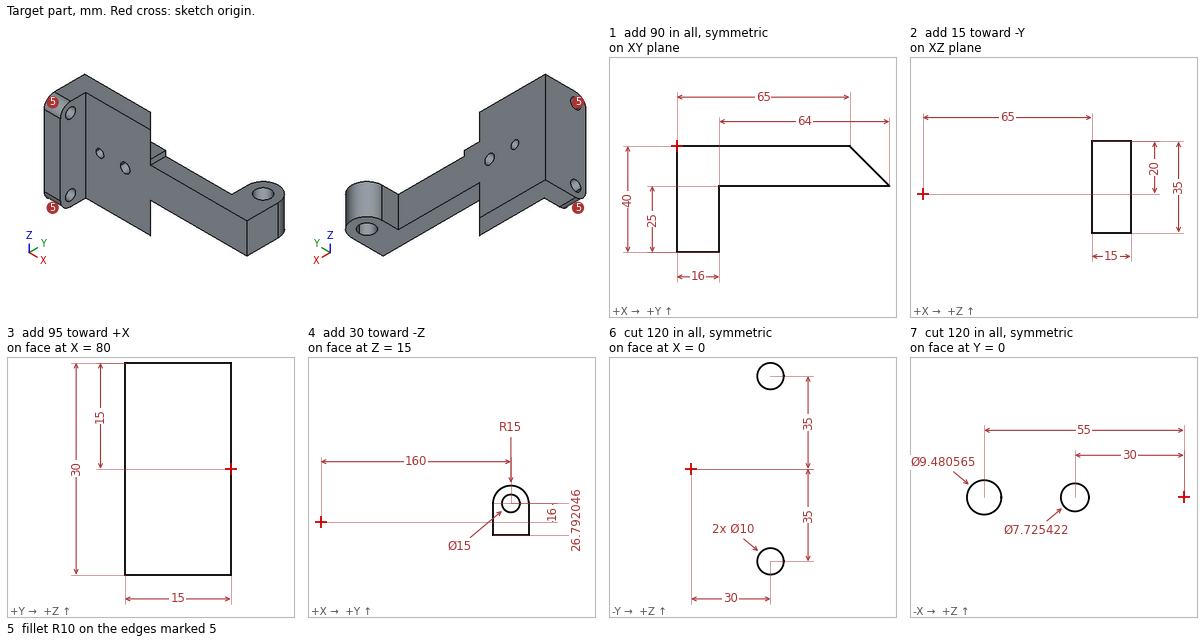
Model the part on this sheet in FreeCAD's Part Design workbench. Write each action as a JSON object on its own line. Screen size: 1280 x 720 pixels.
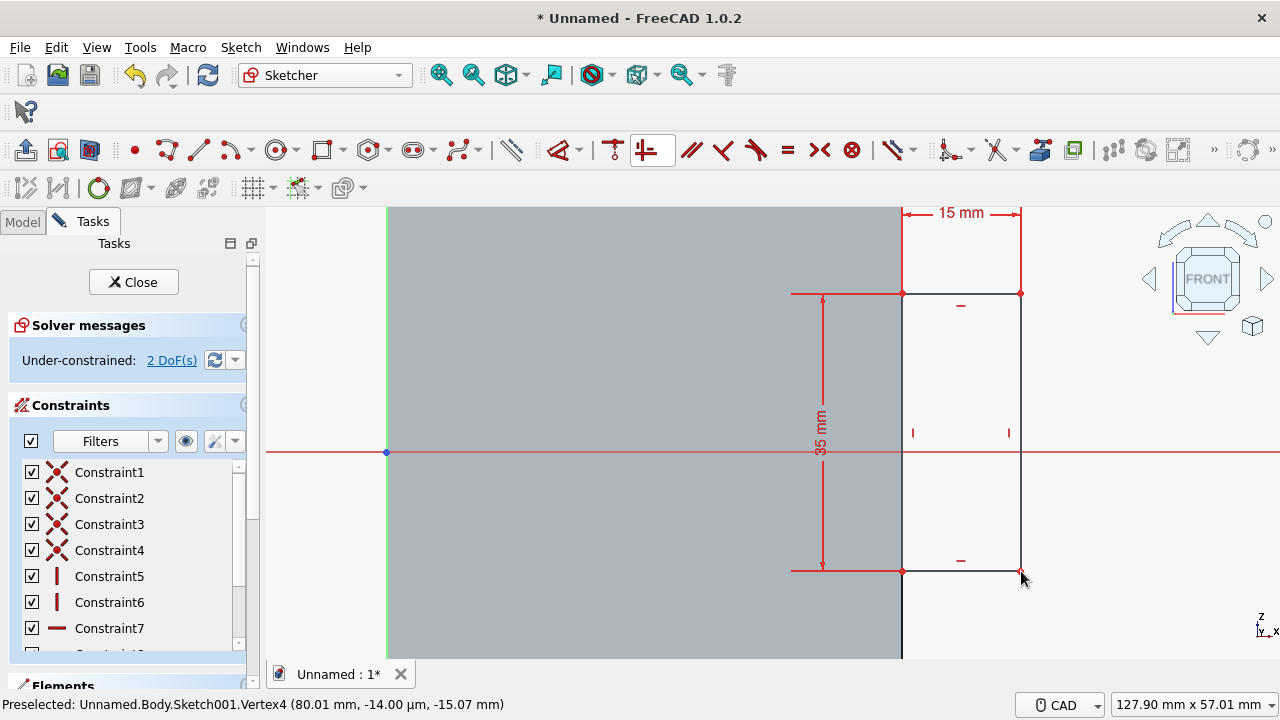
{"action": "left_click", "coordinate": [558, 150]}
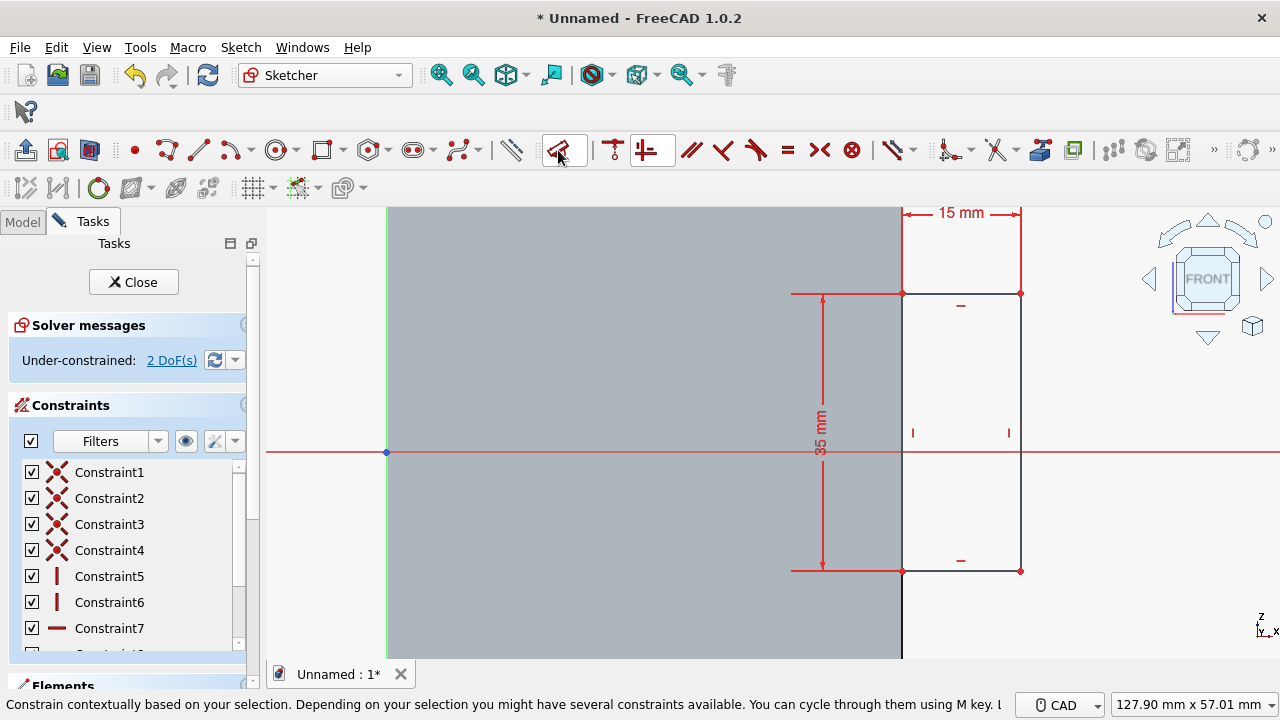
{"action": "left_click", "coordinate": [902, 294]}
{"action": "left_click", "coordinate": [644, 260]}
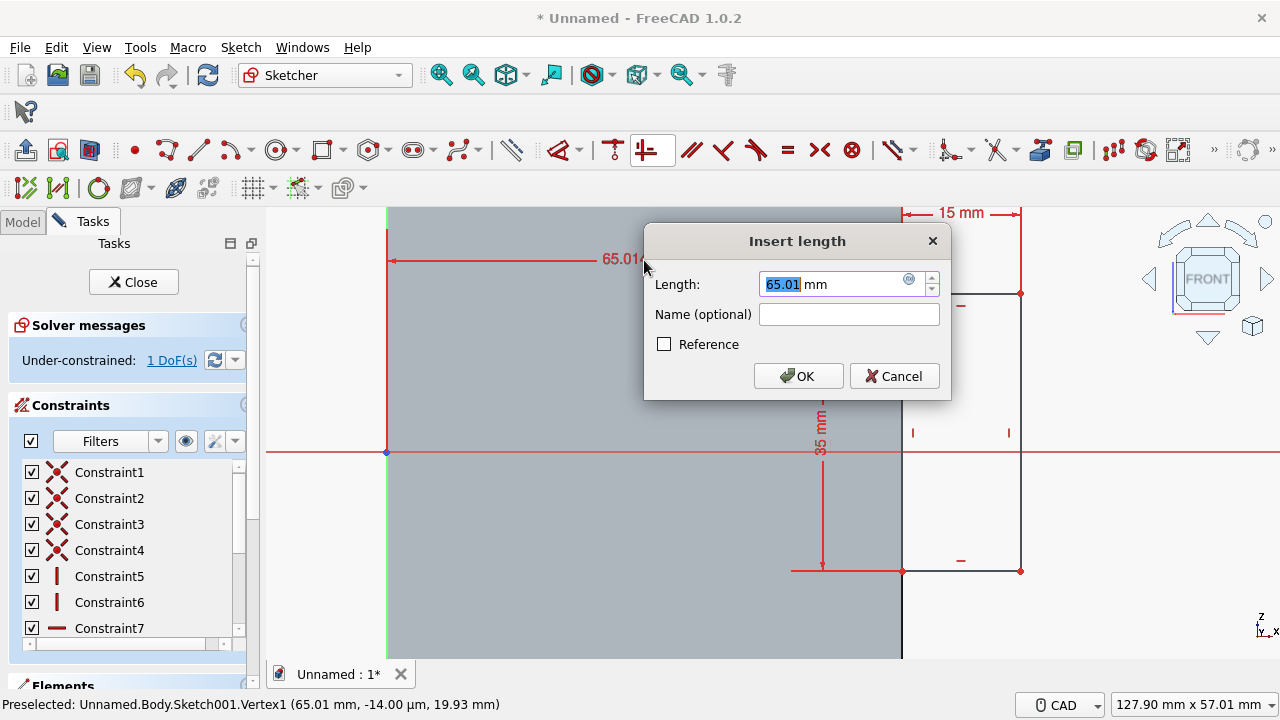
{"action": "type", "text": "65"}
{"action": "key", "text": "Return"}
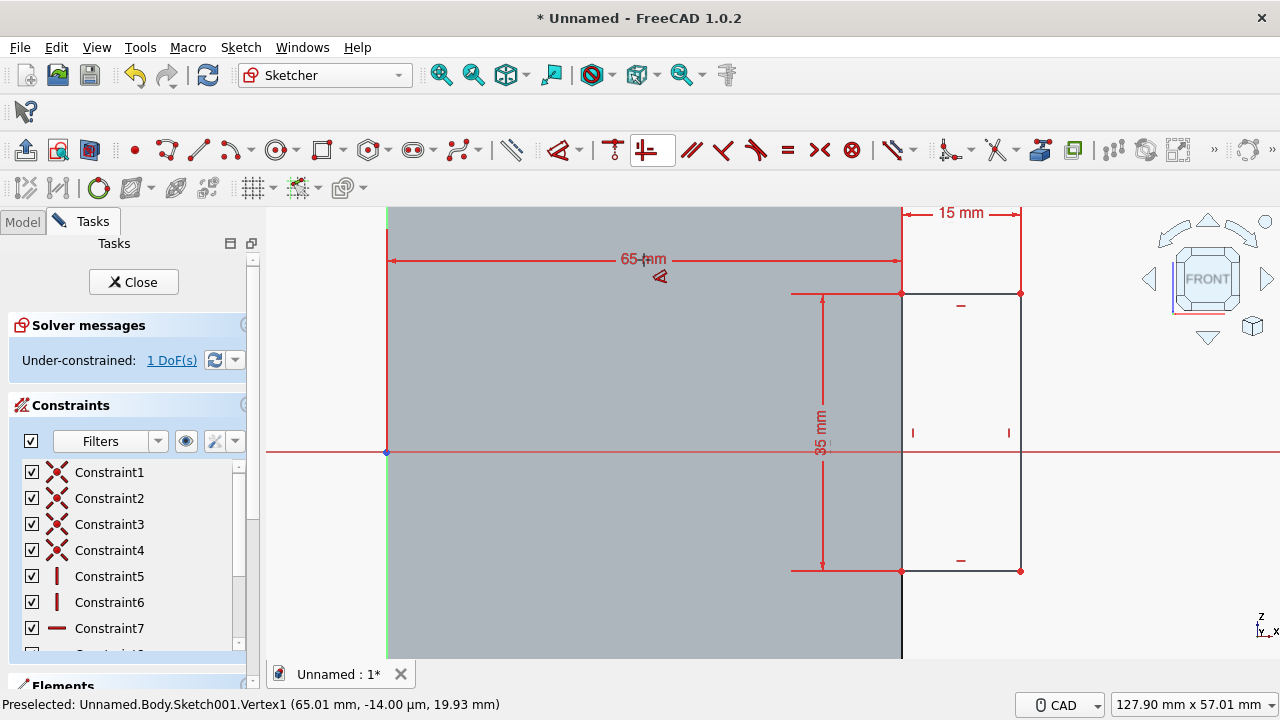
{"action": "left_click", "coordinate": [902, 294]}
{"action": "left_click", "coordinate": [353, 373]}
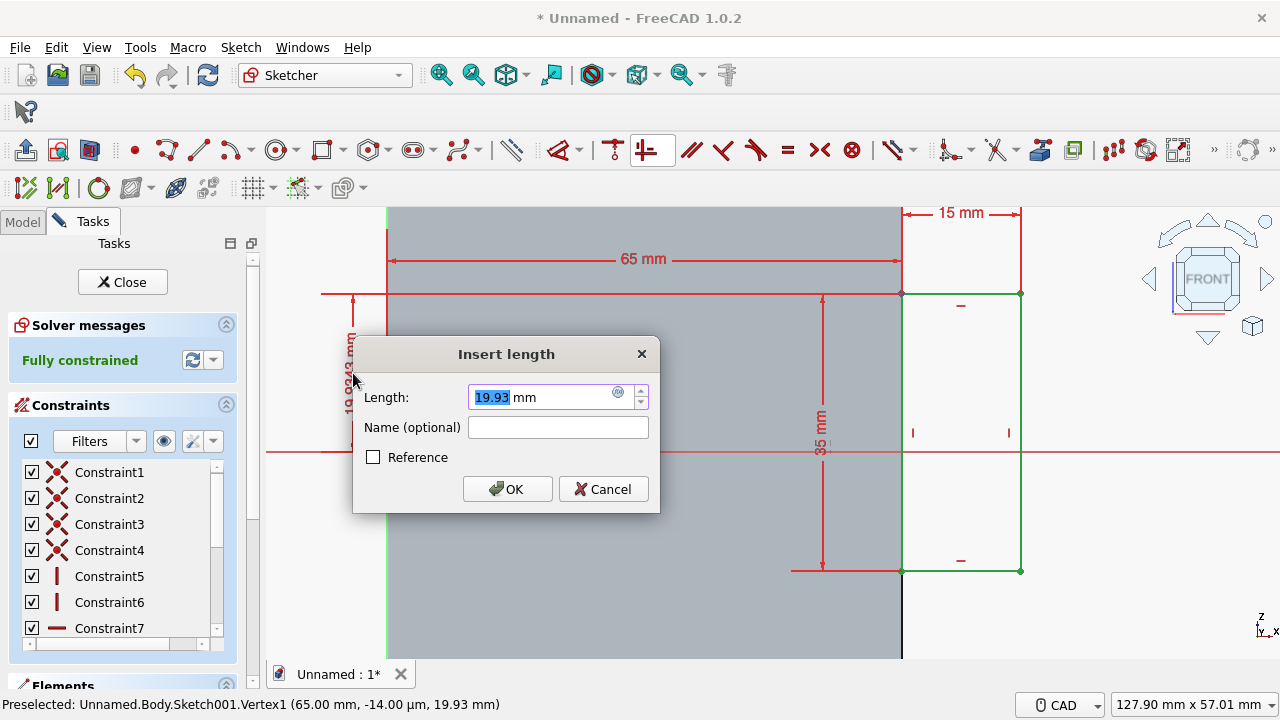
{"action": "type", "text": "20"}
{"action": "key", "text": "Return"}
{"action": "key", "text": "Escape"}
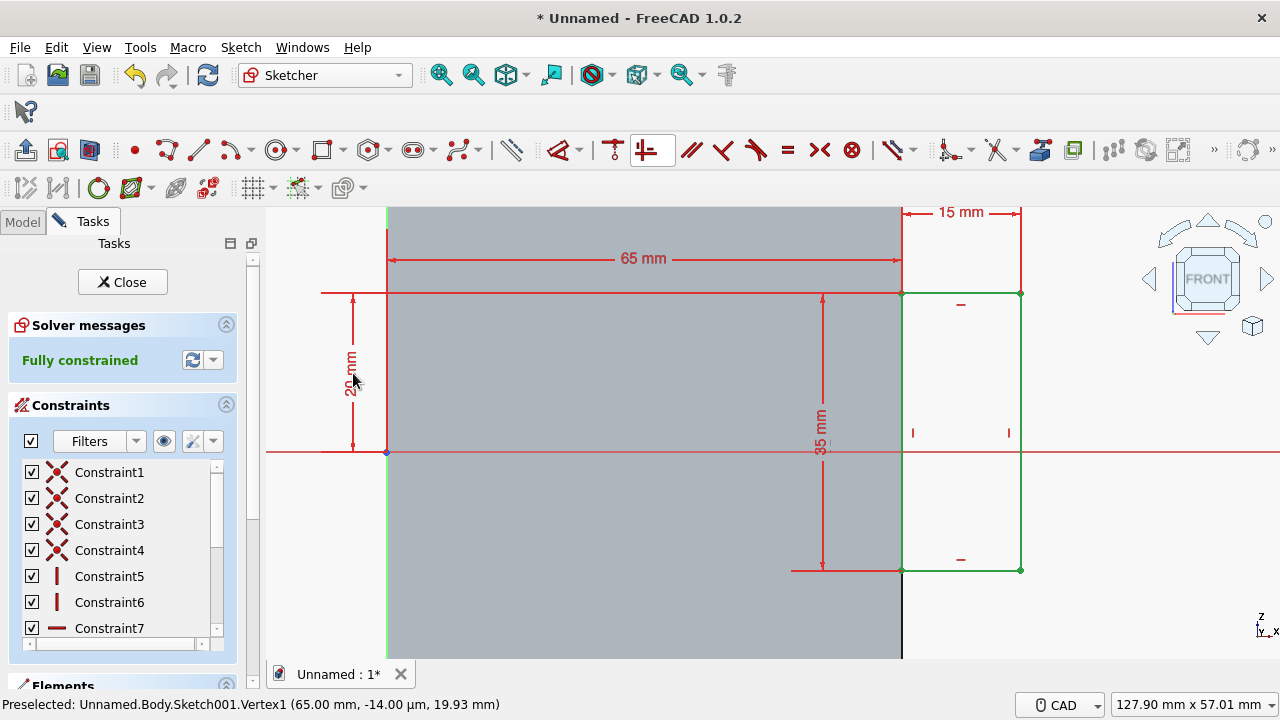
{"action": "left_click", "coordinate": [123, 282]}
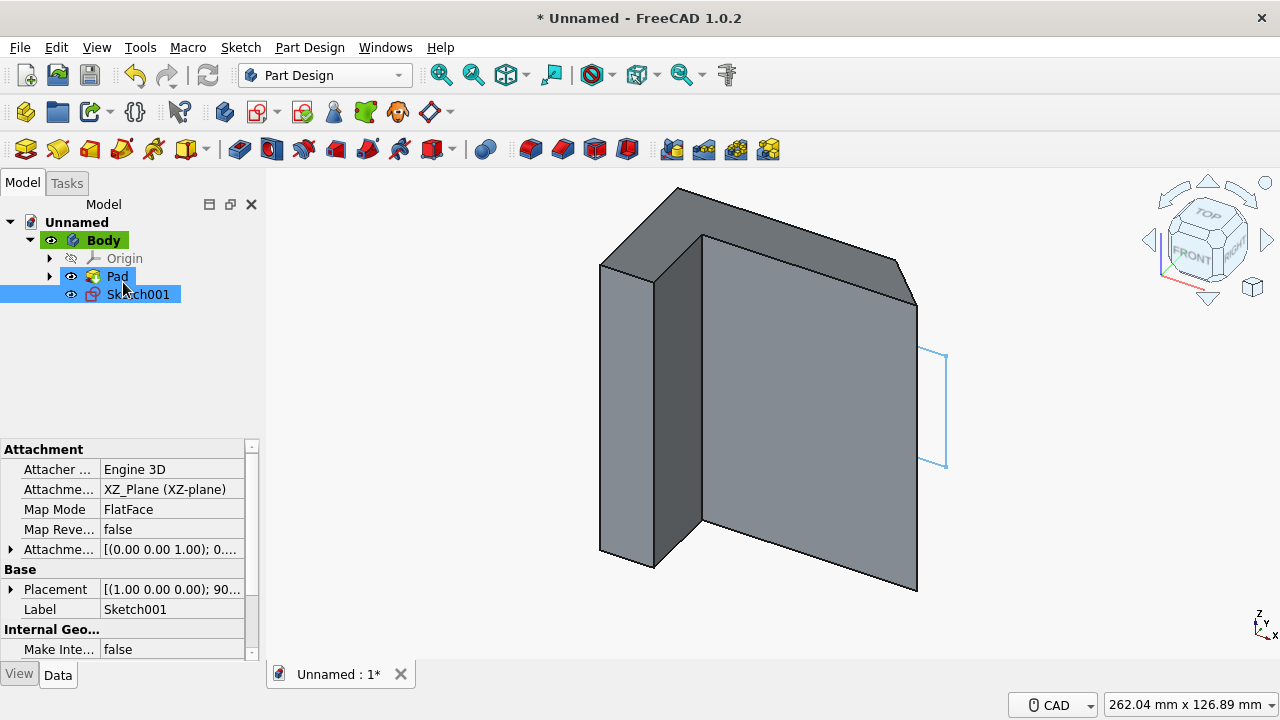
{"action": "left_click", "coordinate": [26, 150]}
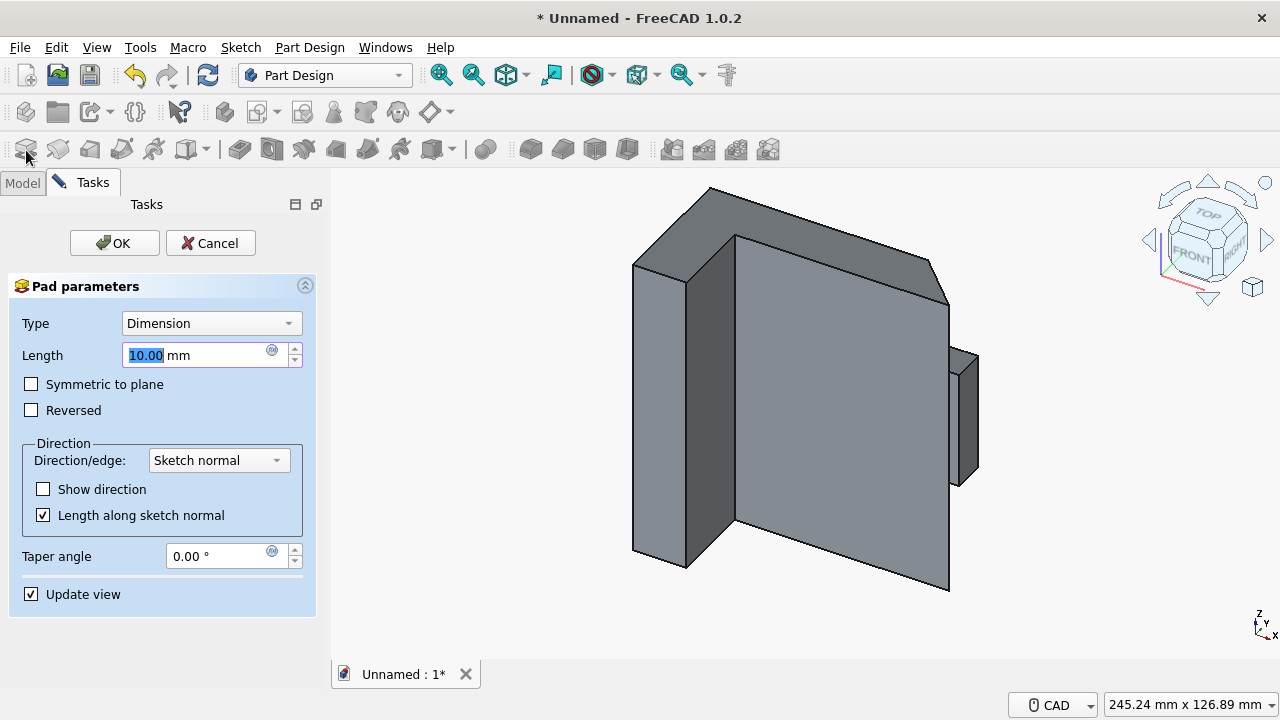
{"action": "type", "text": "15"}
{"action": "key", "text": "Tab"}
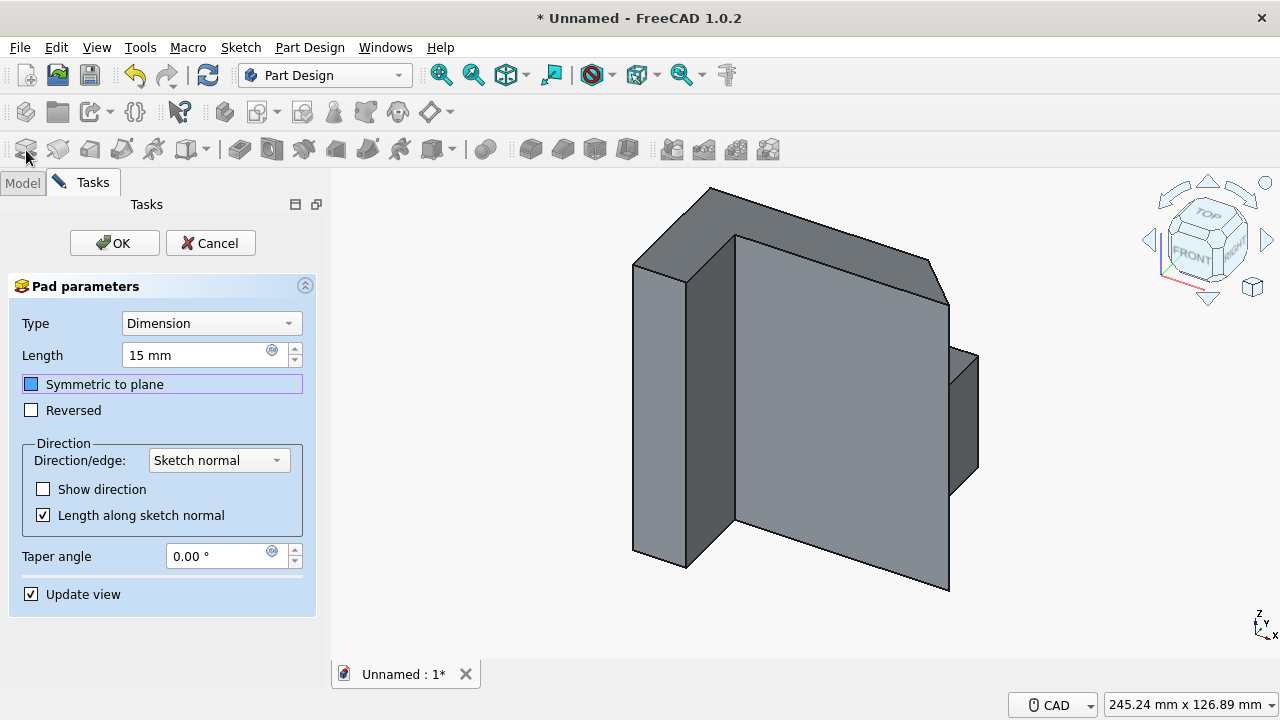
{"action": "left_click", "coordinate": [115, 243]}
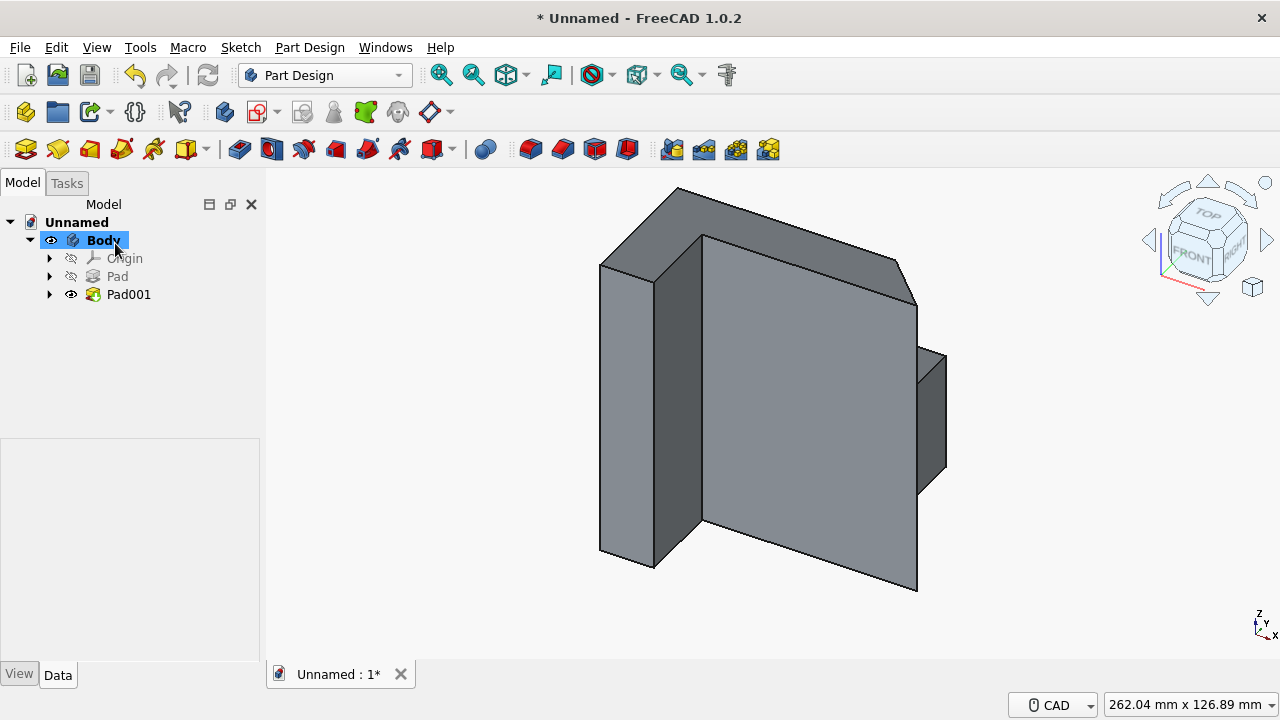
{"action": "left_click", "coordinate": [931, 393]}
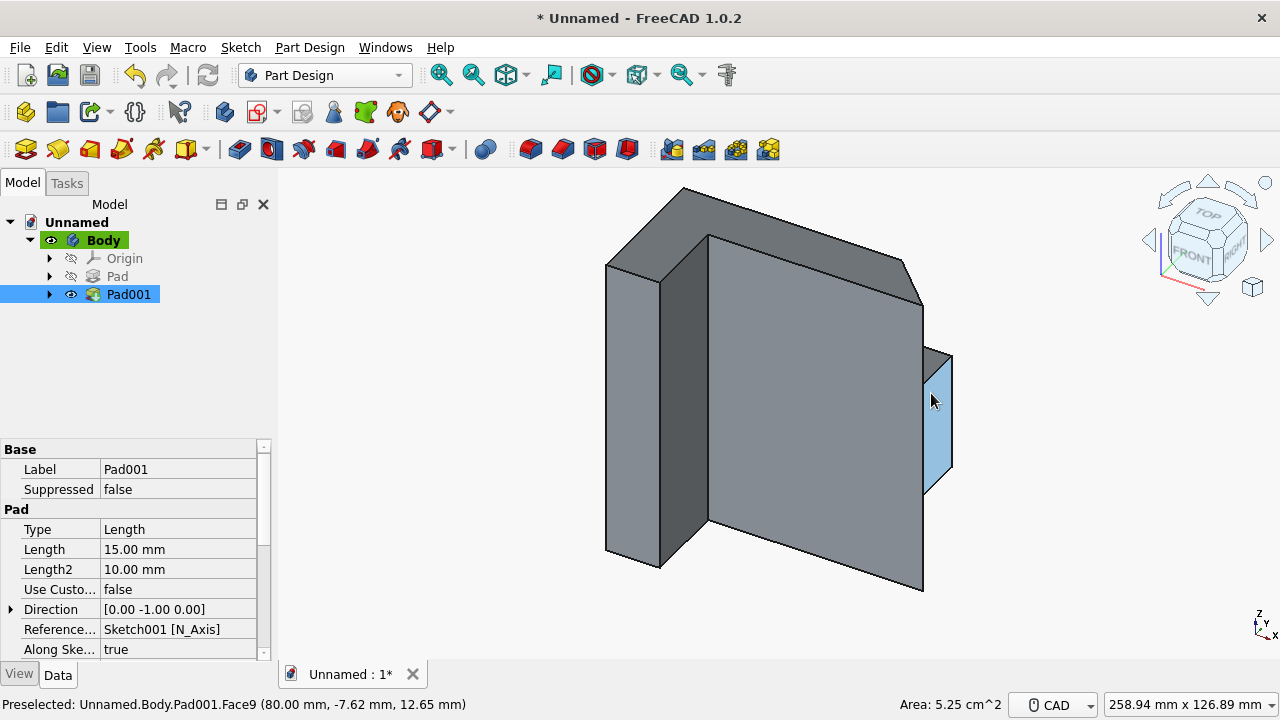
{"action": "left_click", "coordinate": [258, 112]}